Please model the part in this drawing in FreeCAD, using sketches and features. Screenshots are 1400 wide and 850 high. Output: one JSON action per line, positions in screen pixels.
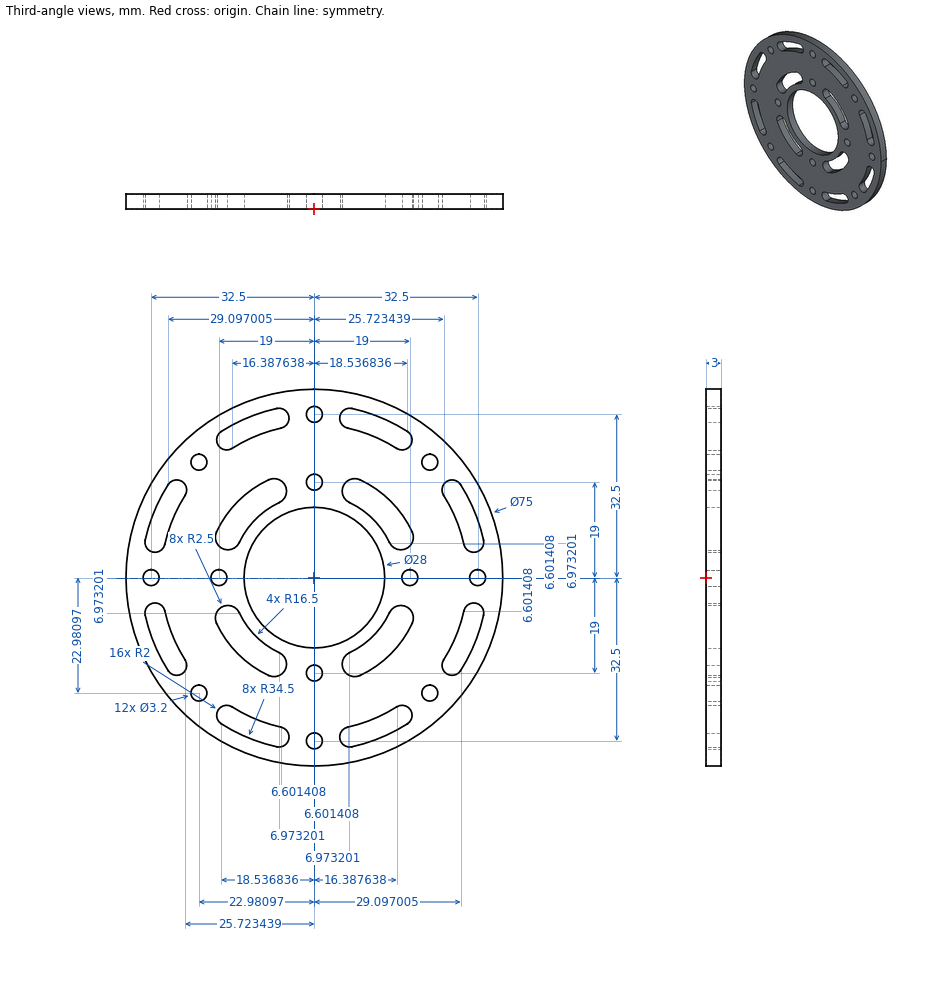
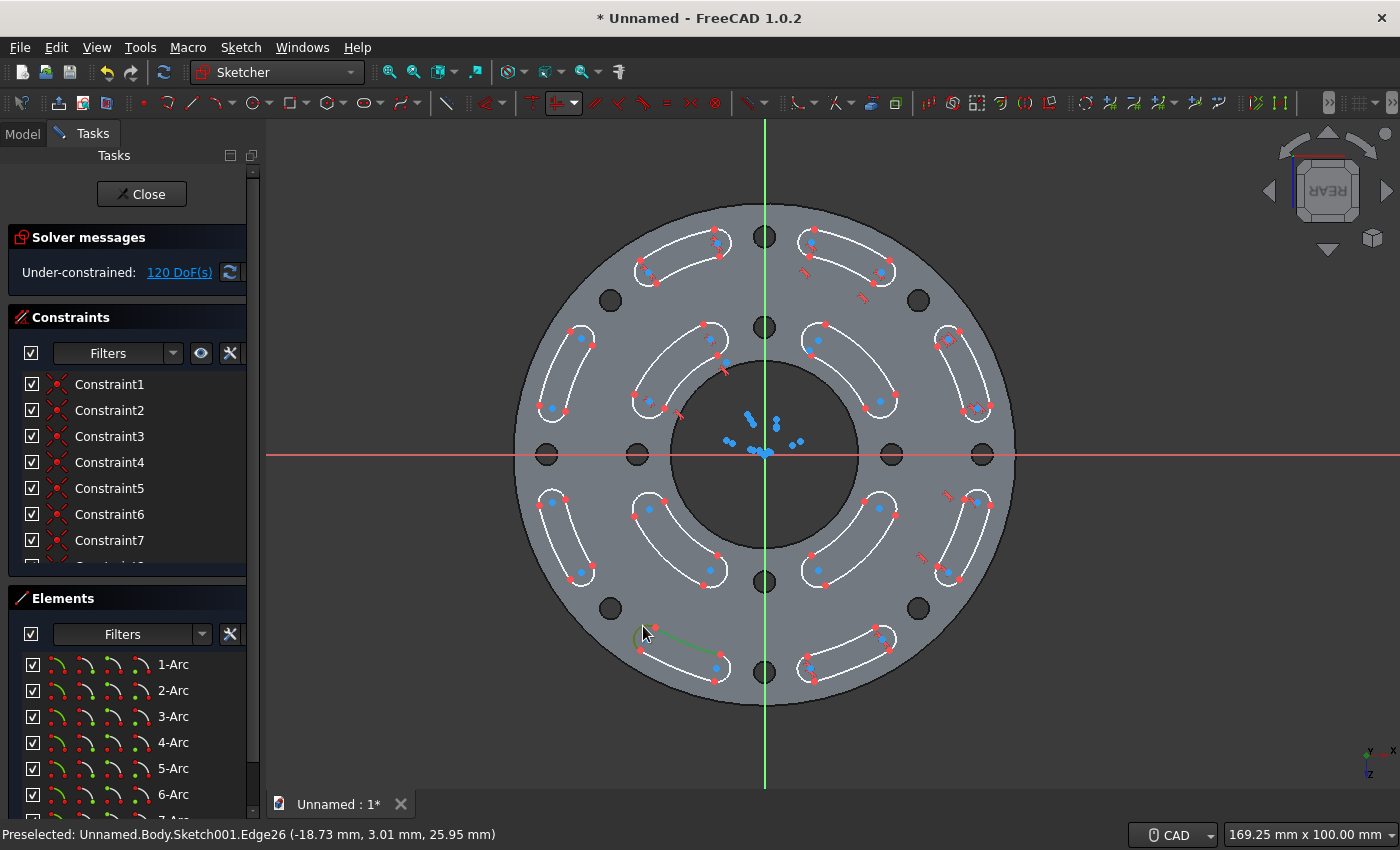
{"action": "left_click", "coordinate": [644, 104]}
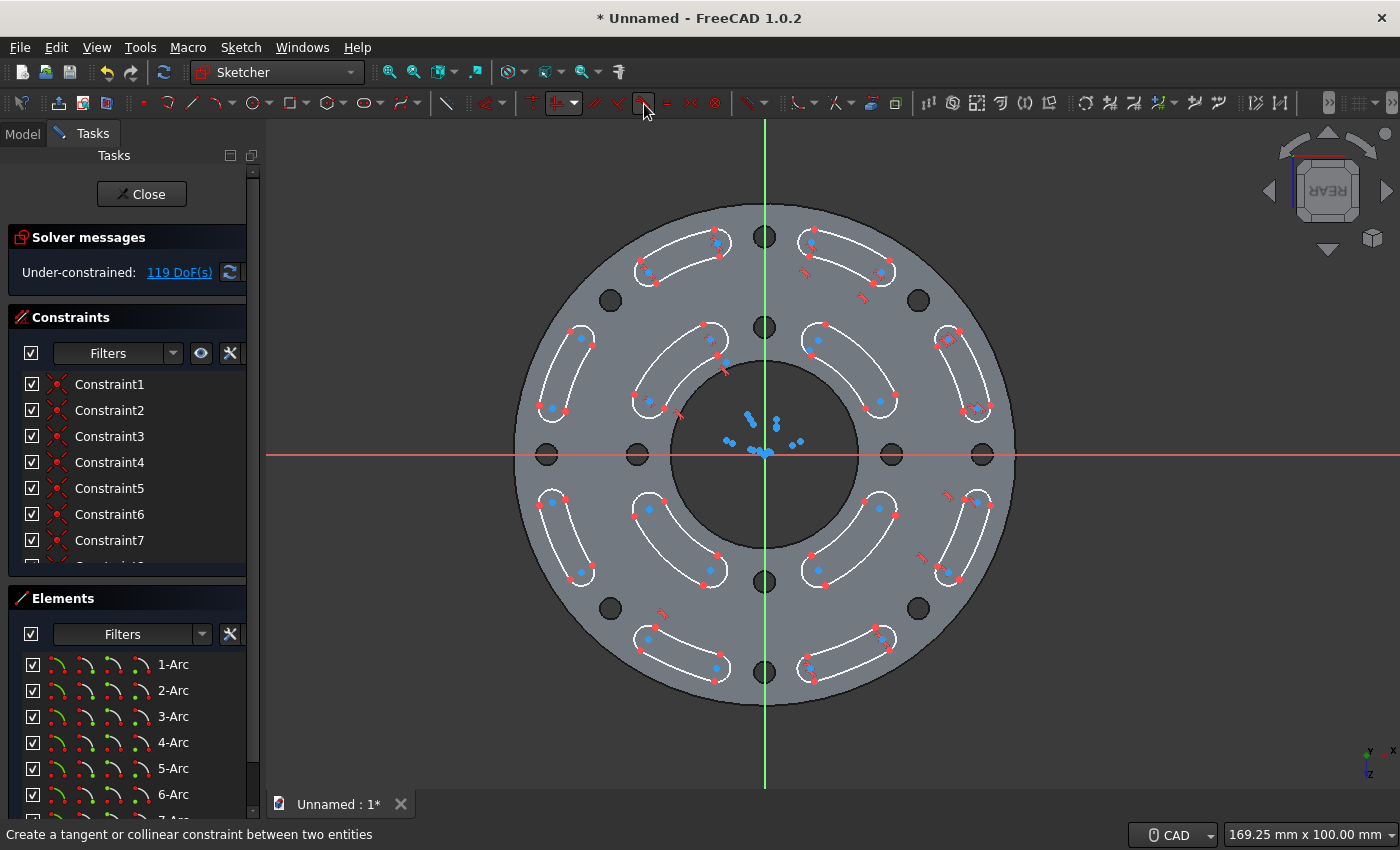
{"action": "left_click", "coordinate": [674, 638]}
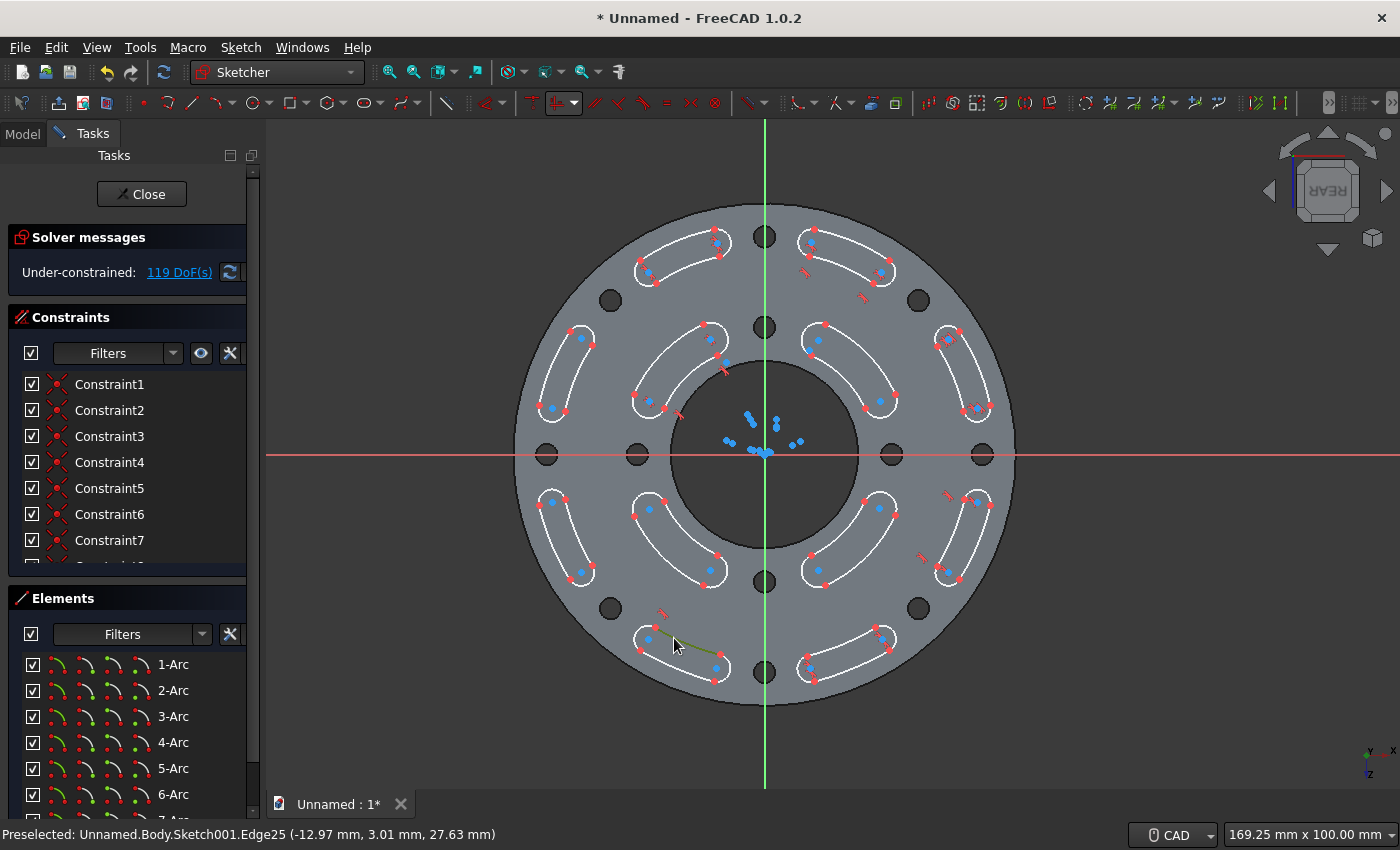
{"action": "left_click", "coordinate": [726, 678]}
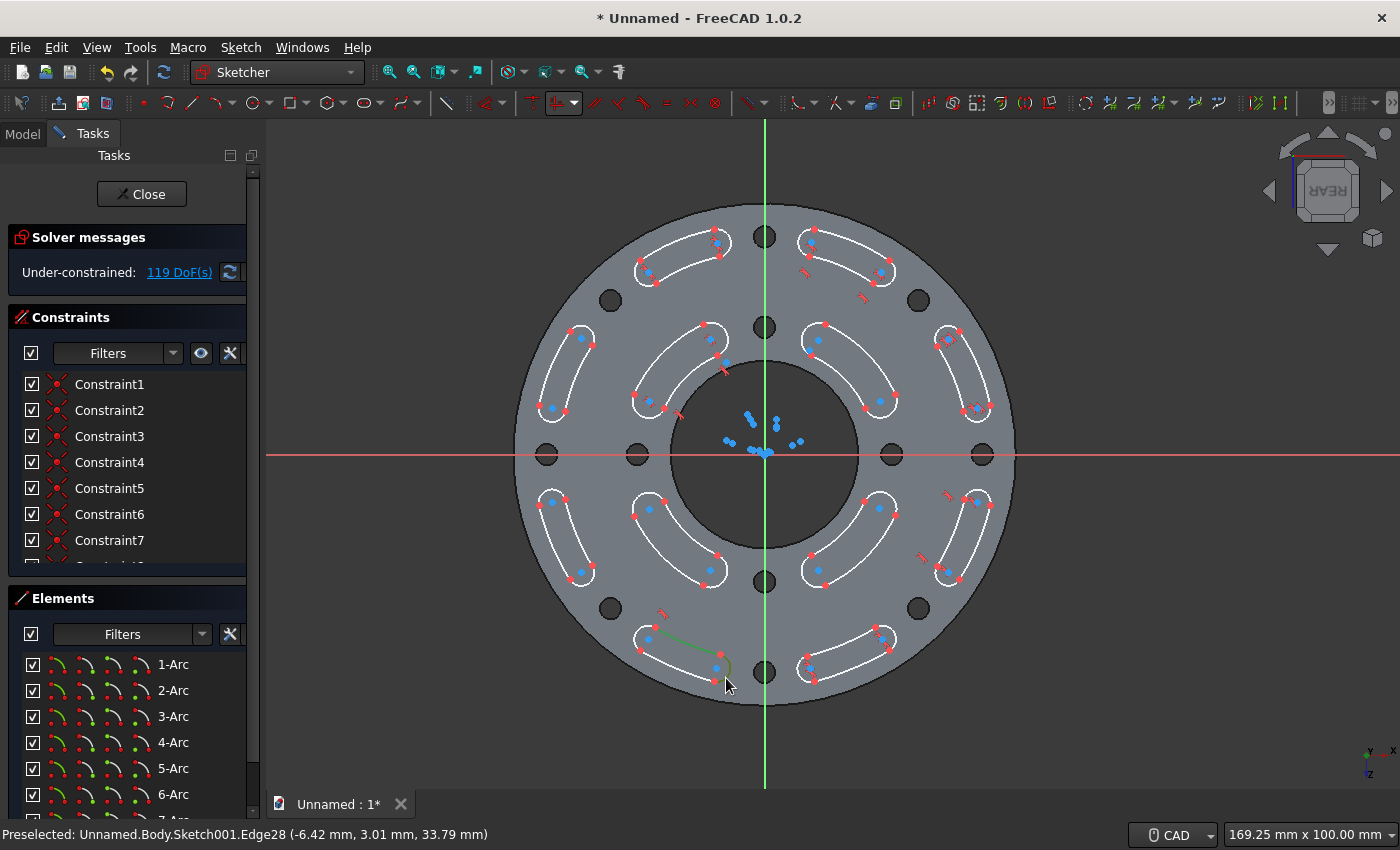
{"action": "left_click", "coordinate": [644, 104]}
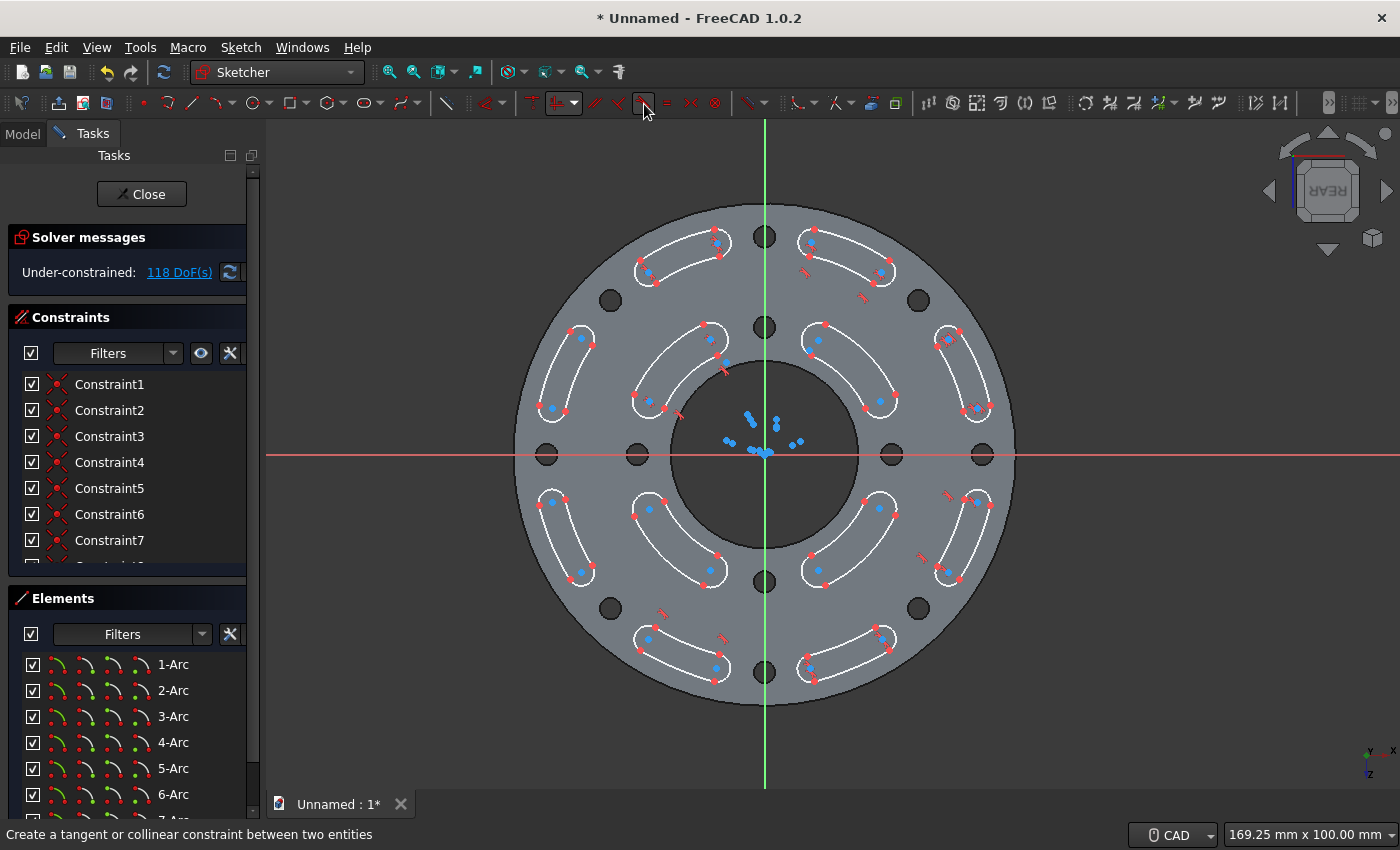
{"action": "left_click", "coordinate": [643, 627]}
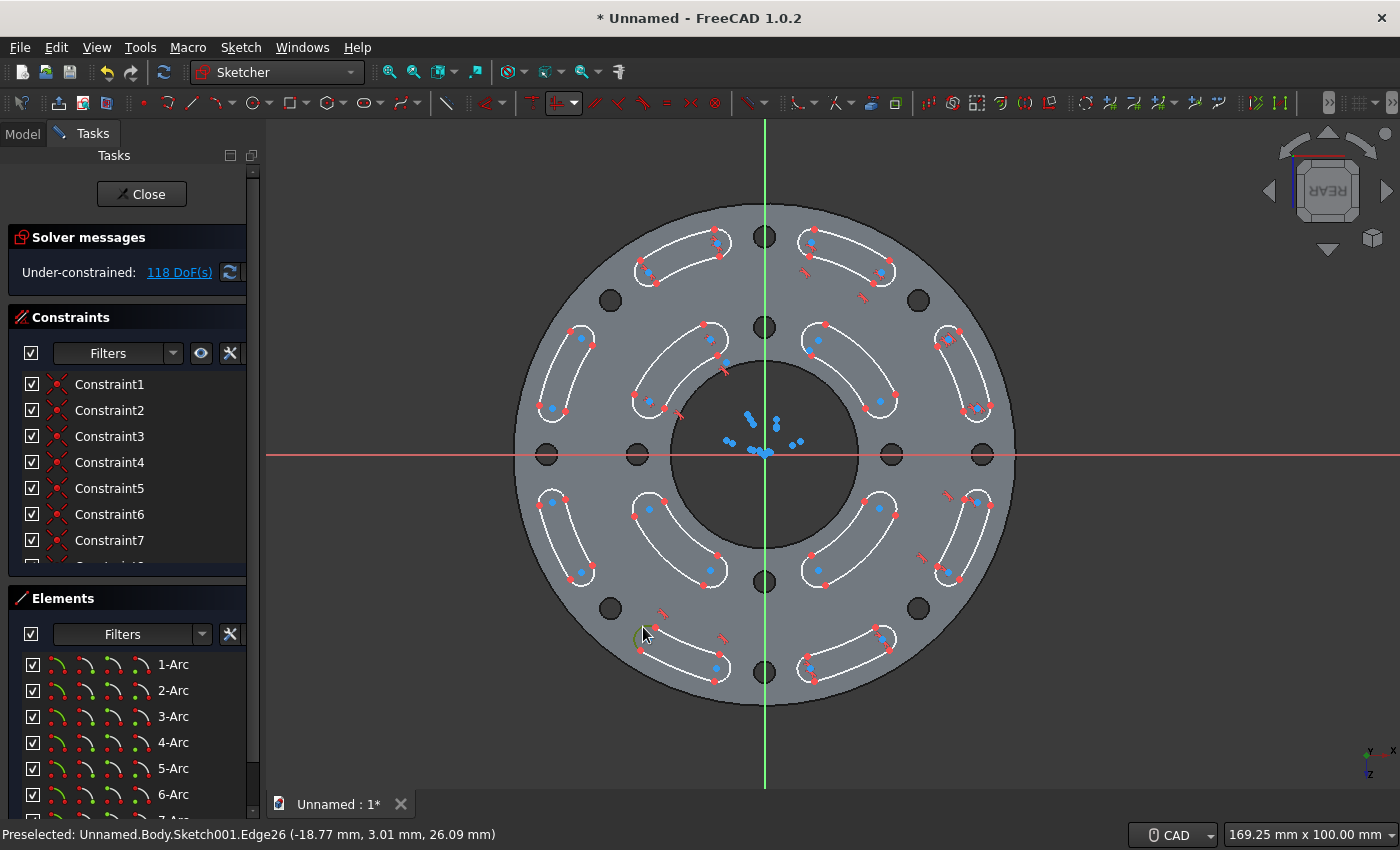
{"action": "left_click", "coordinate": [661, 662]}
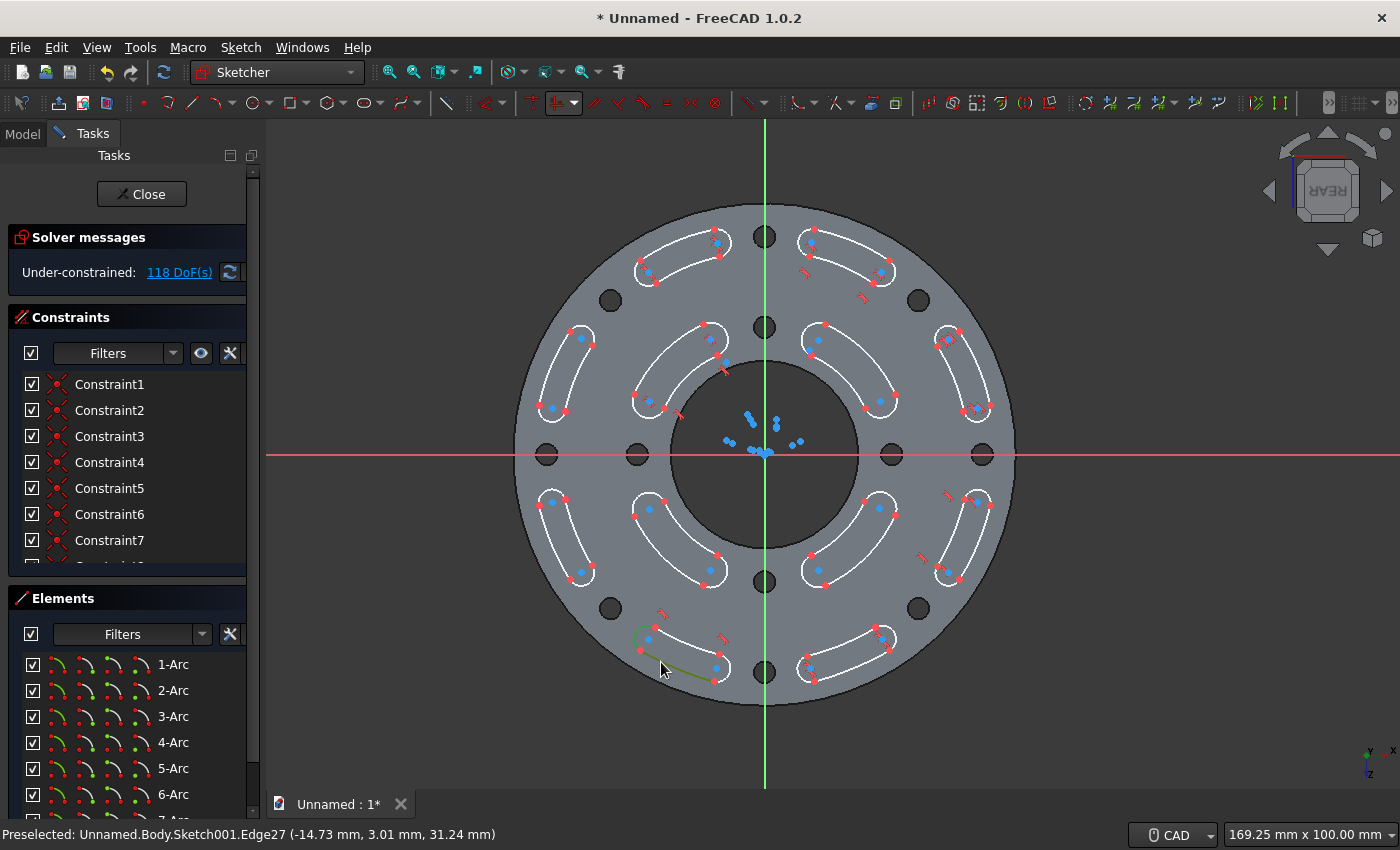
{"action": "left_click", "coordinate": [644, 104]}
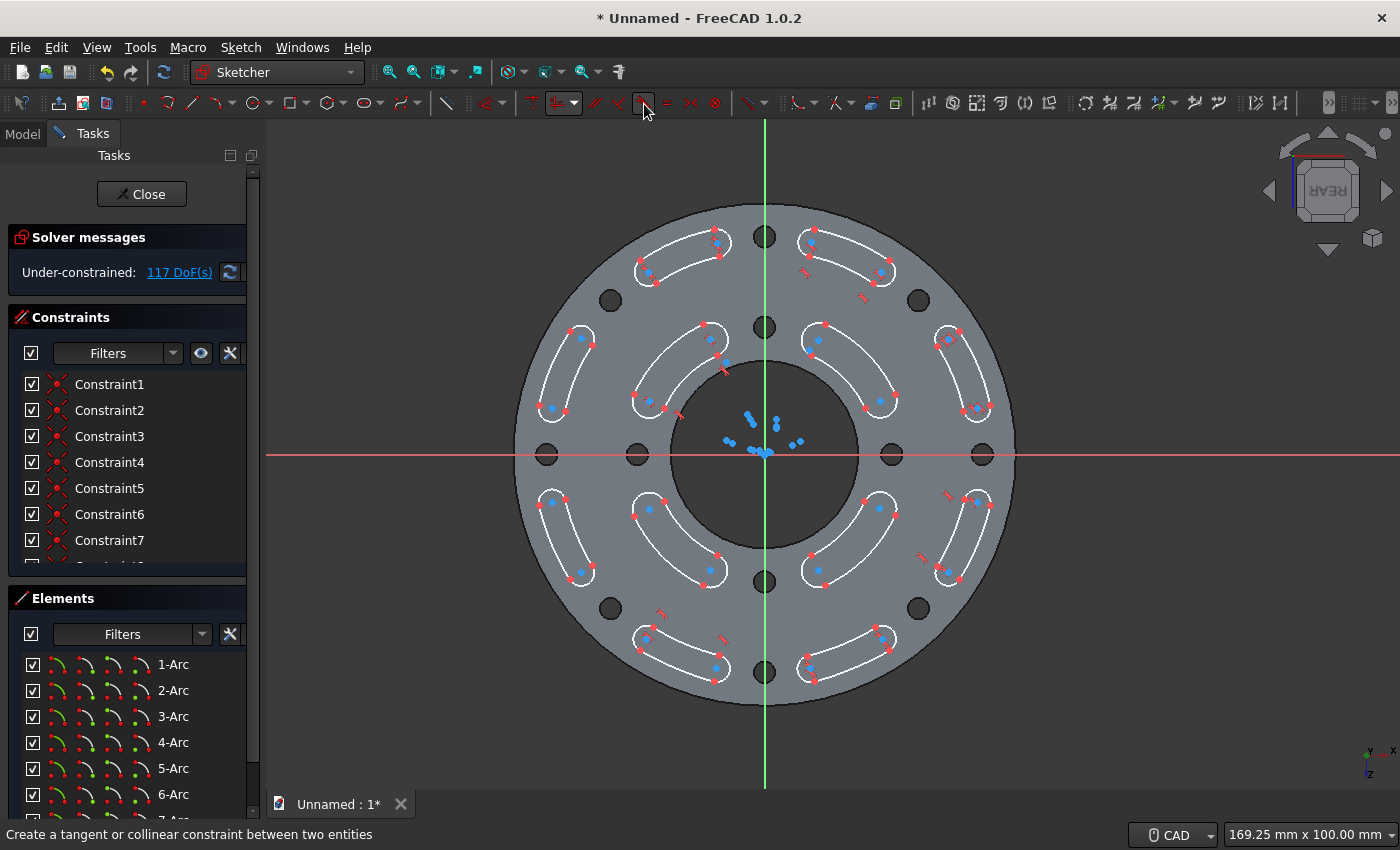
{"action": "left_click", "coordinate": [662, 662]}